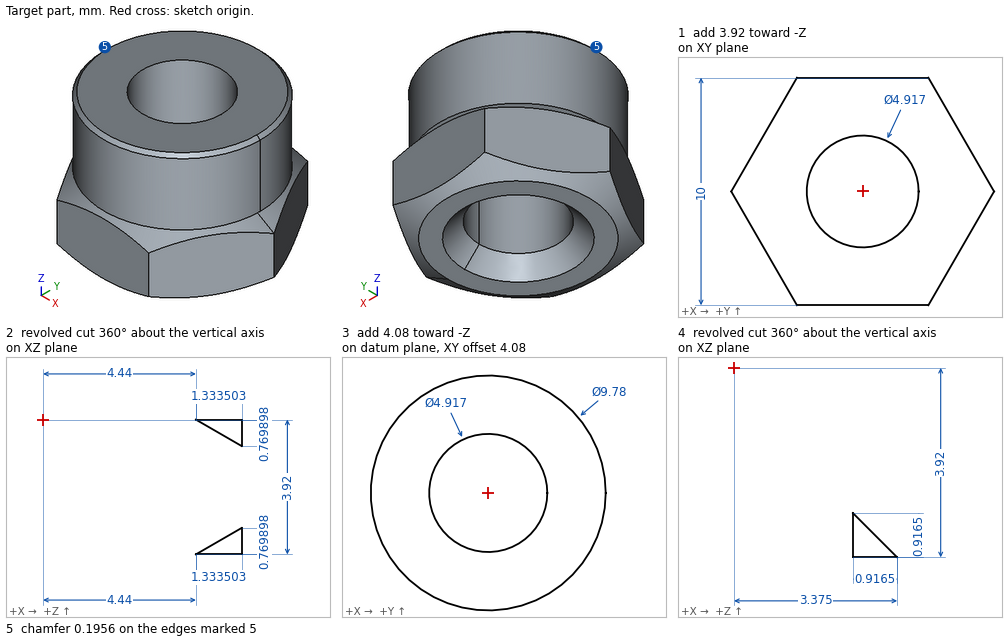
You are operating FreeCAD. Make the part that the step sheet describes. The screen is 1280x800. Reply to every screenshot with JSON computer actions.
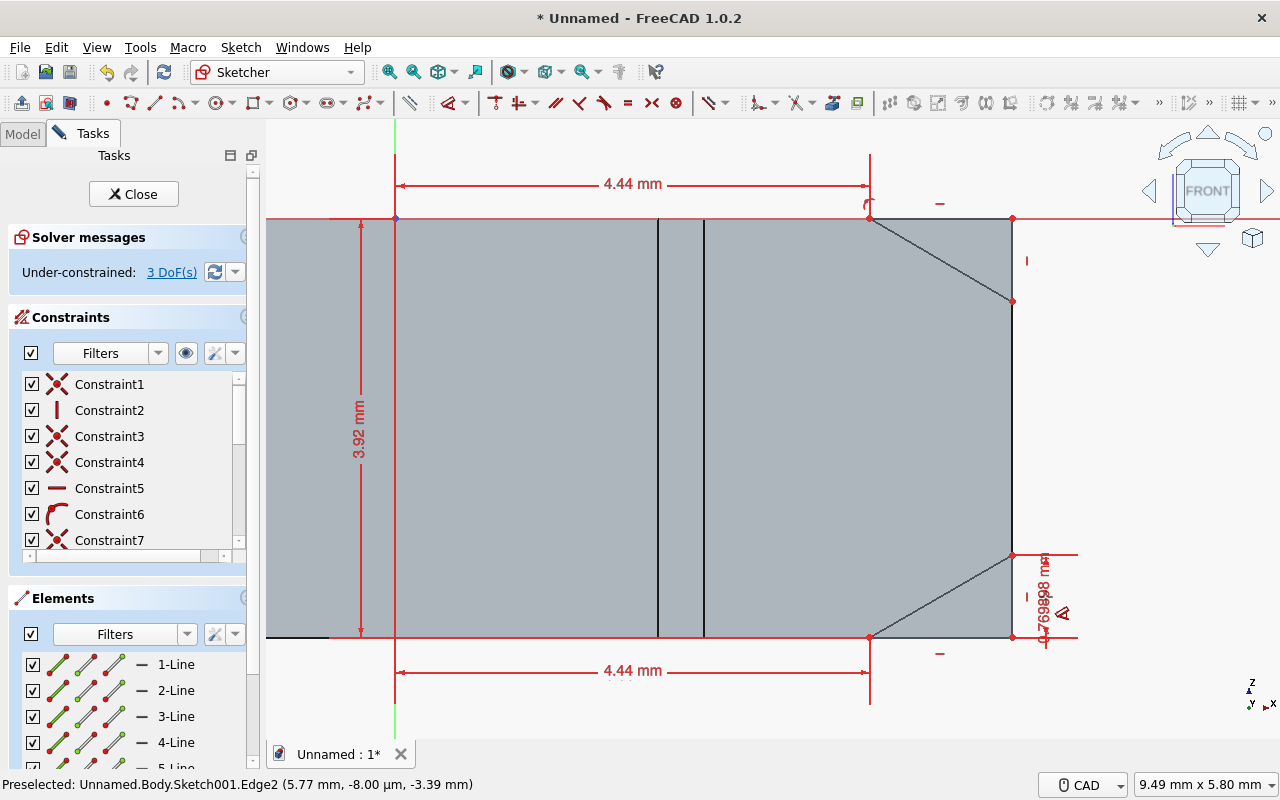
{"action": "left_click", "coordinate": [969, 638]}
{"action": "left_click", "coordinate": [941, 672]}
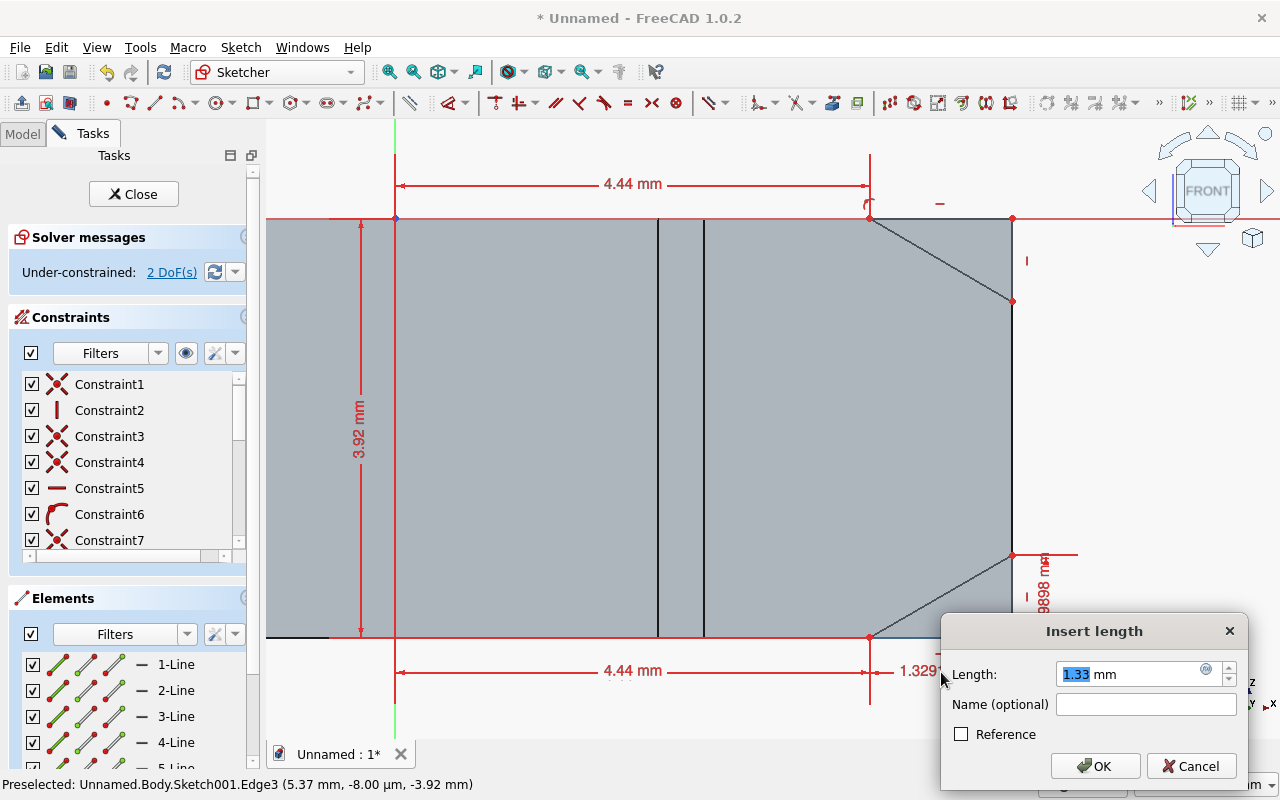
{"action": "type", "text": "1.333503"}
{"action": "key", "text": "Return"}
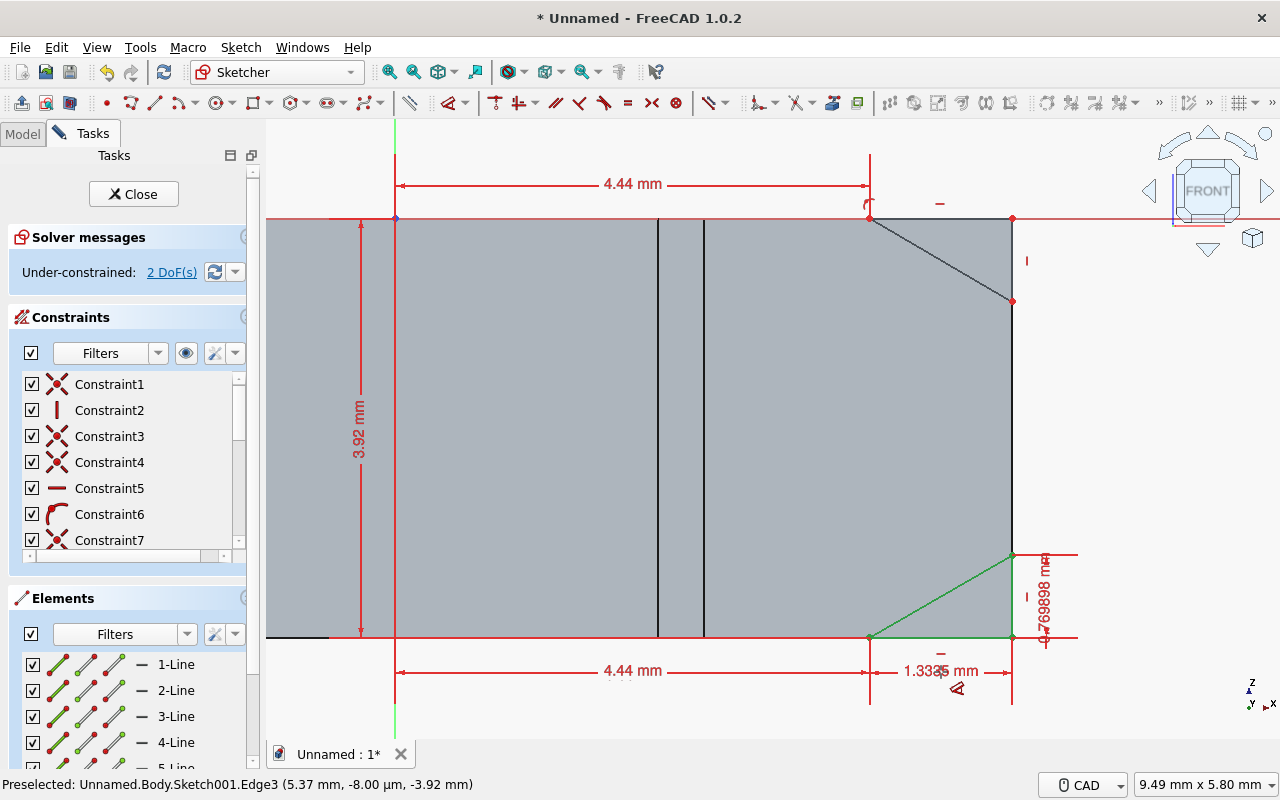
{"action": "left_click", "coordinate": [913, 219]}
{"action": "left_click", "coordinate": [941, 185]}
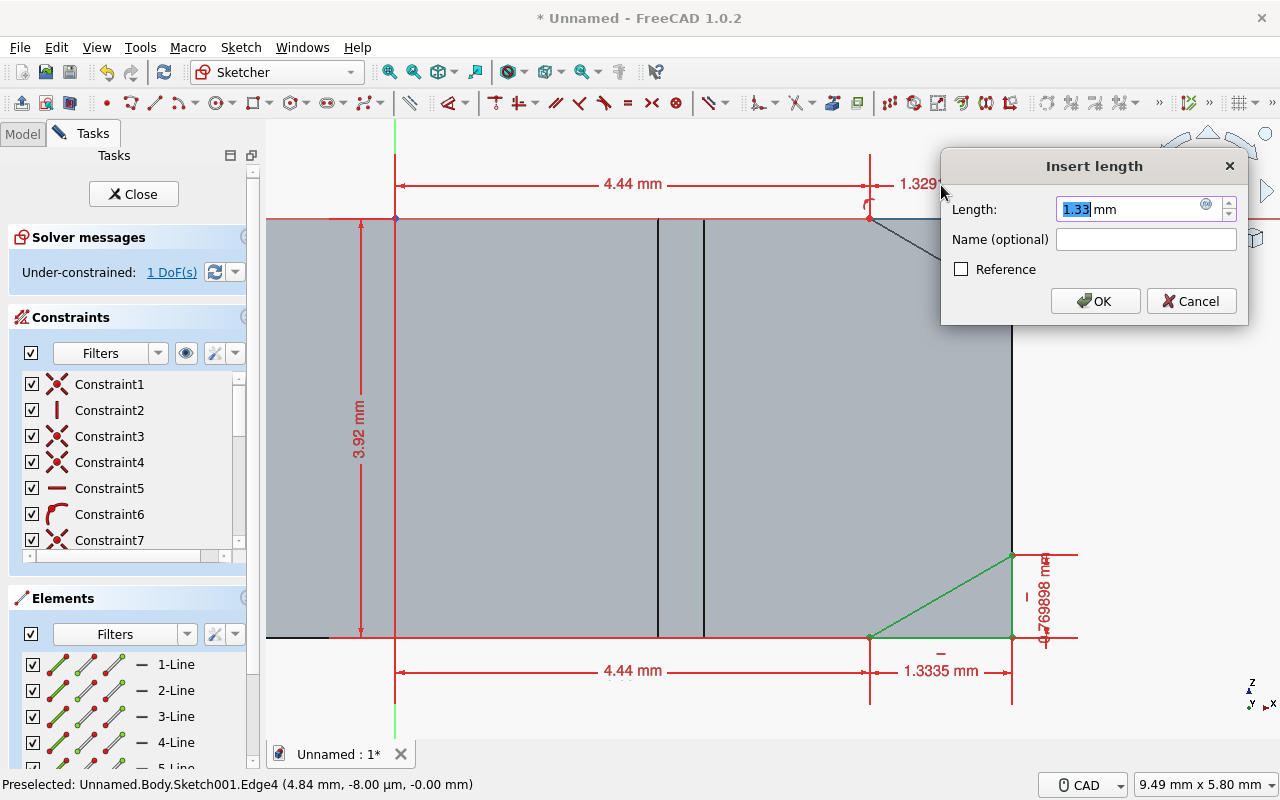
{"action": "type", "text": "1.333503"}
{"action": "key", "text": "Return"}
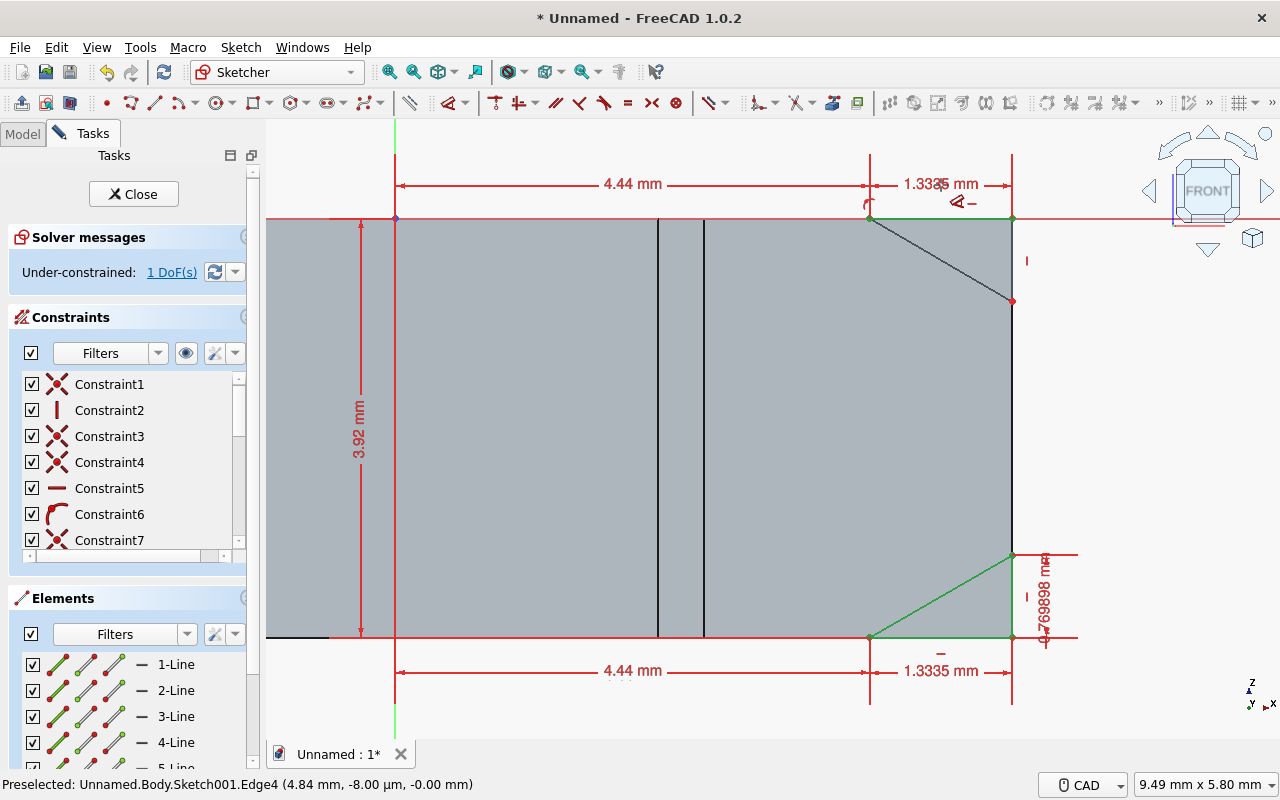
{"action": "left_click", "coordinate": [1012, 244]}
{"action": "left_click", "coordinate": [1046, 260]}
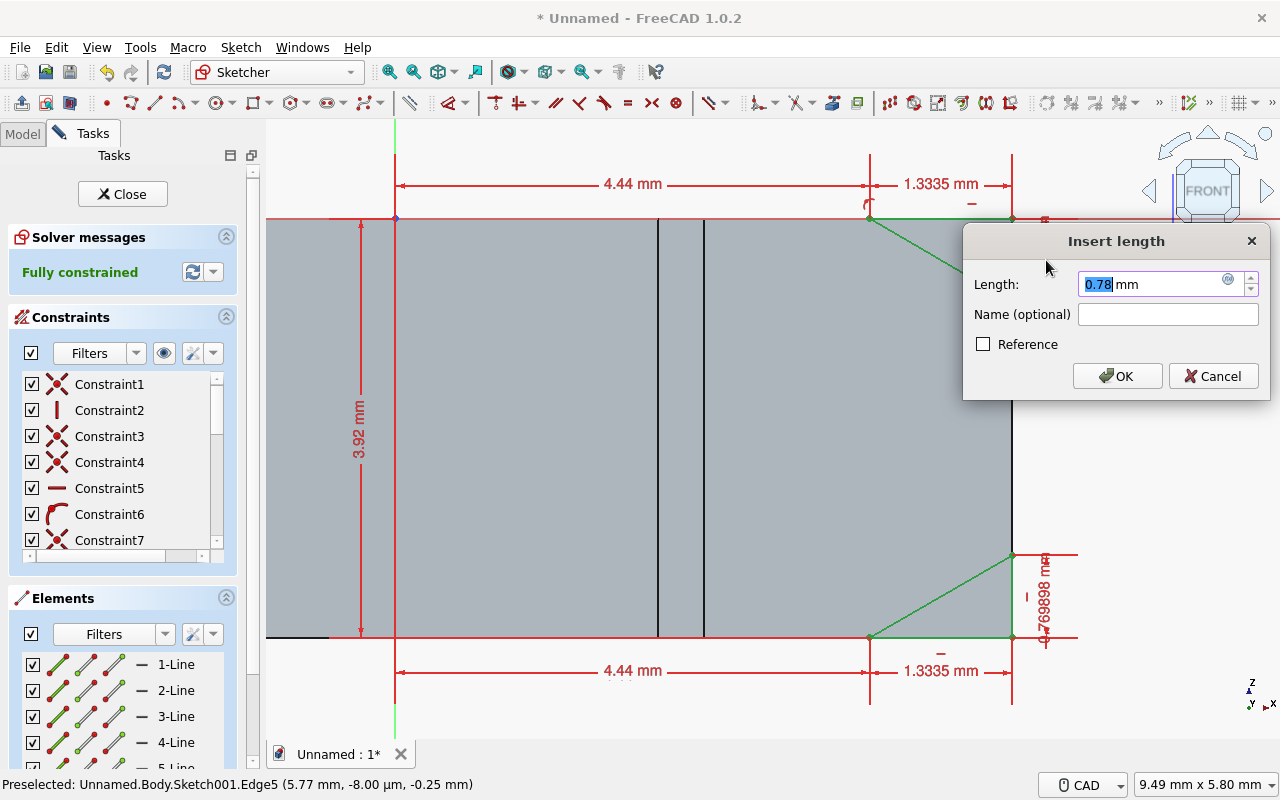
{"action": "type", "text": "0.769898"}
{"action": "key", "text": "Return"}
{"action": "key", "text": "Escape"}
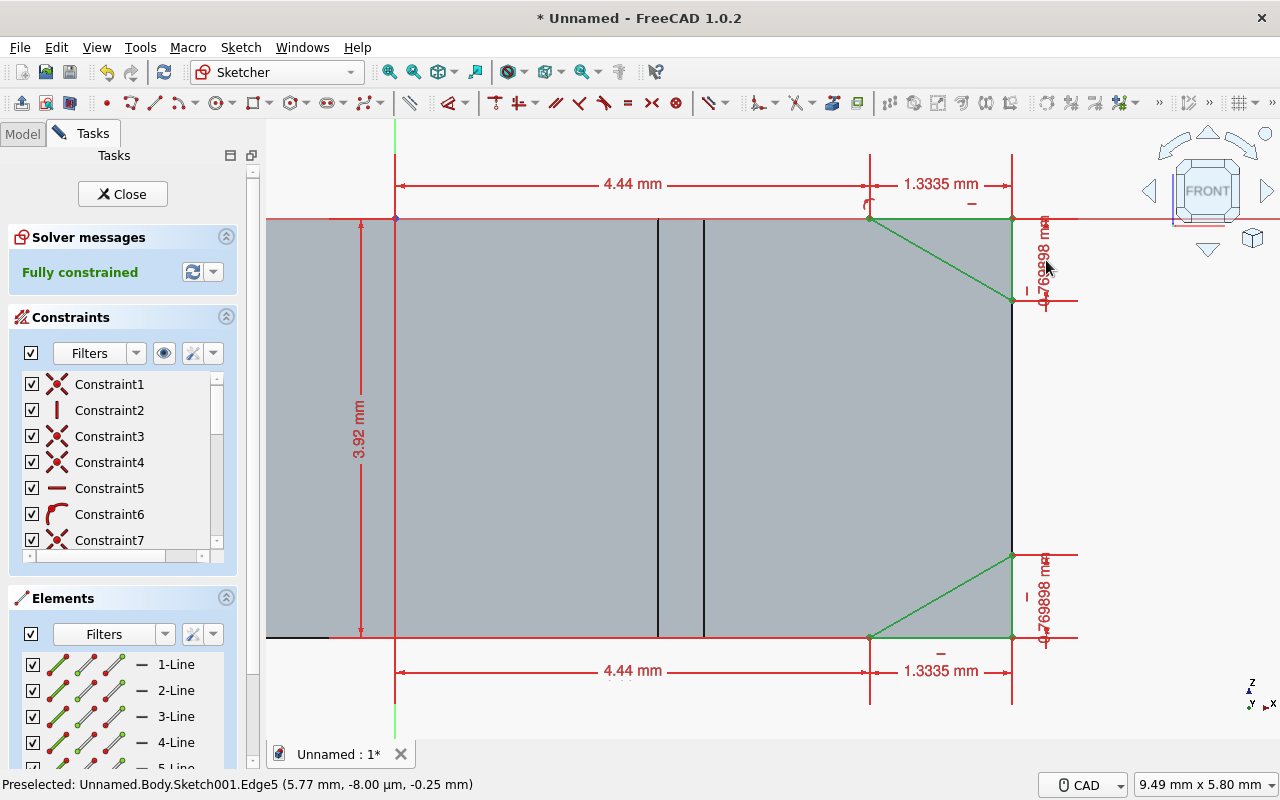
{"action": "left_click", "coordinate": [123, 194]}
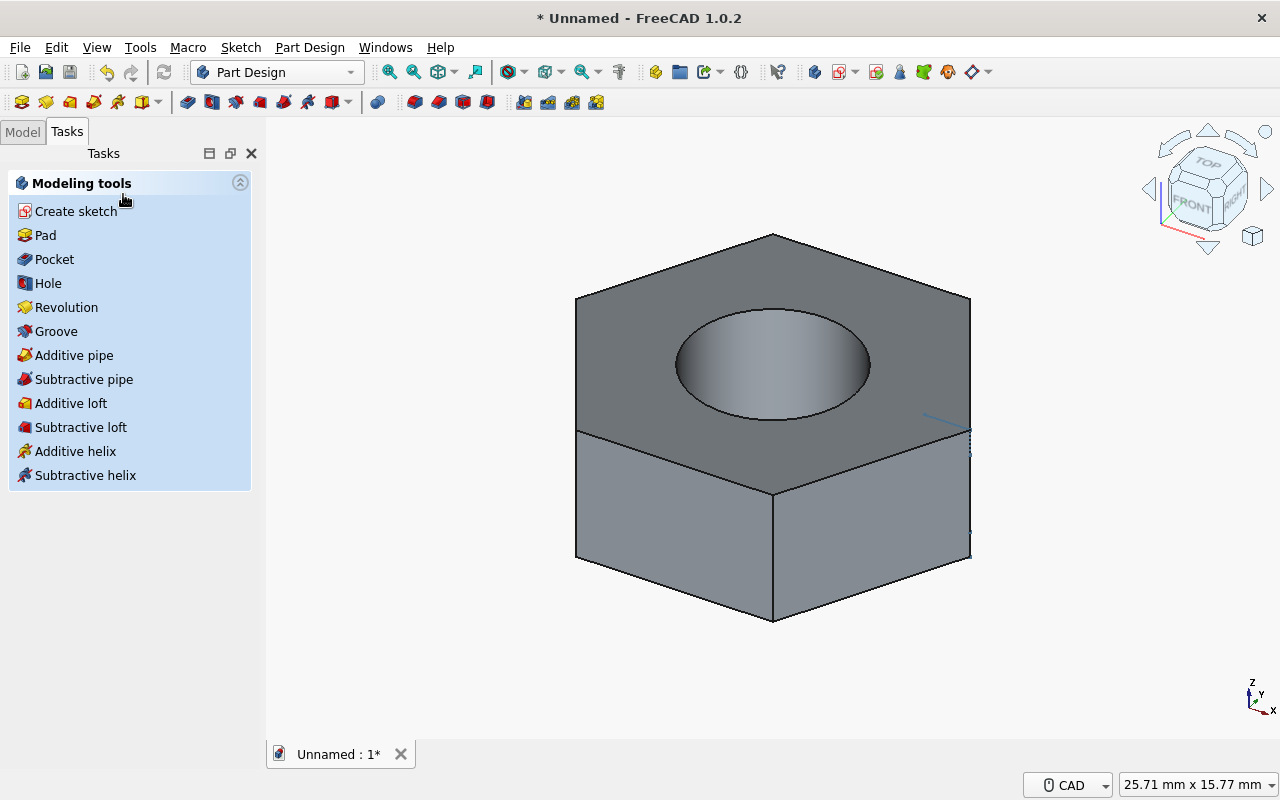
{"action": "left_click", "coordinate": [236, 102]}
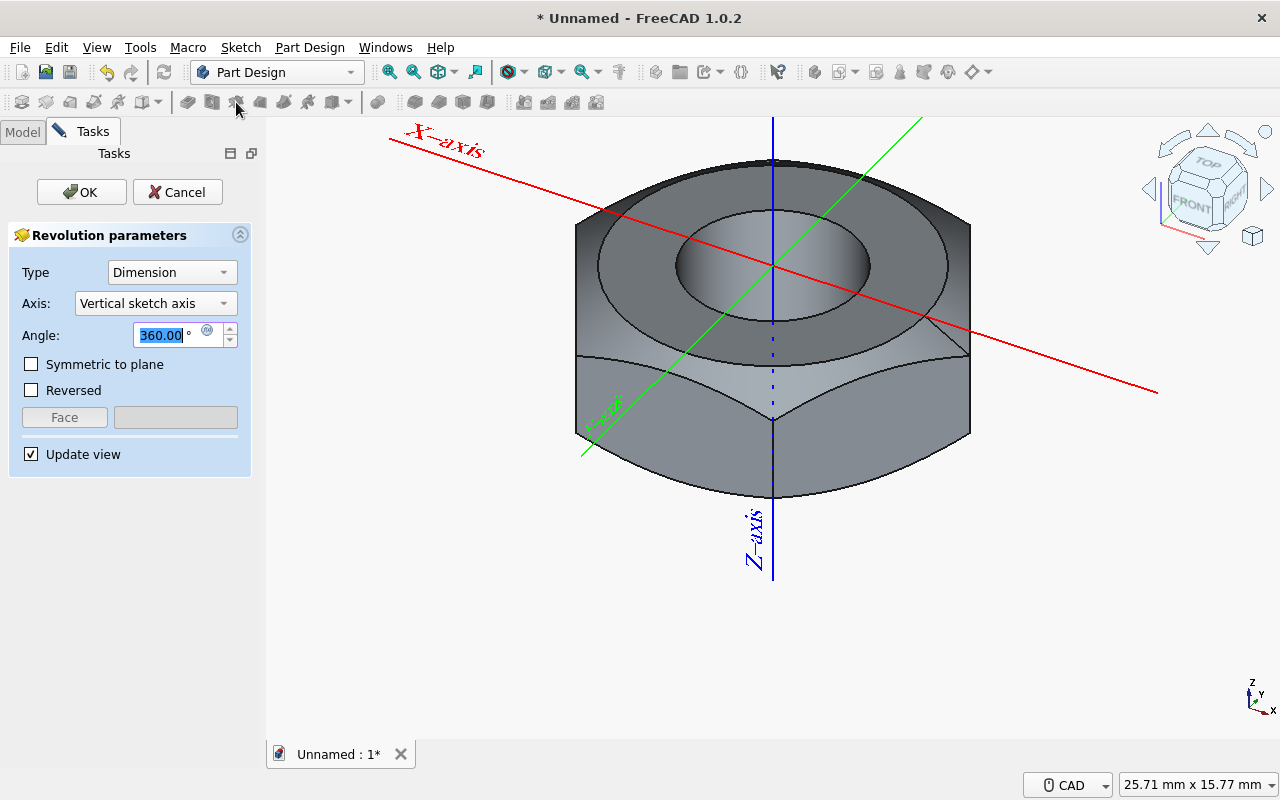
{"action": "left_click", "coordinate": [82, 192]}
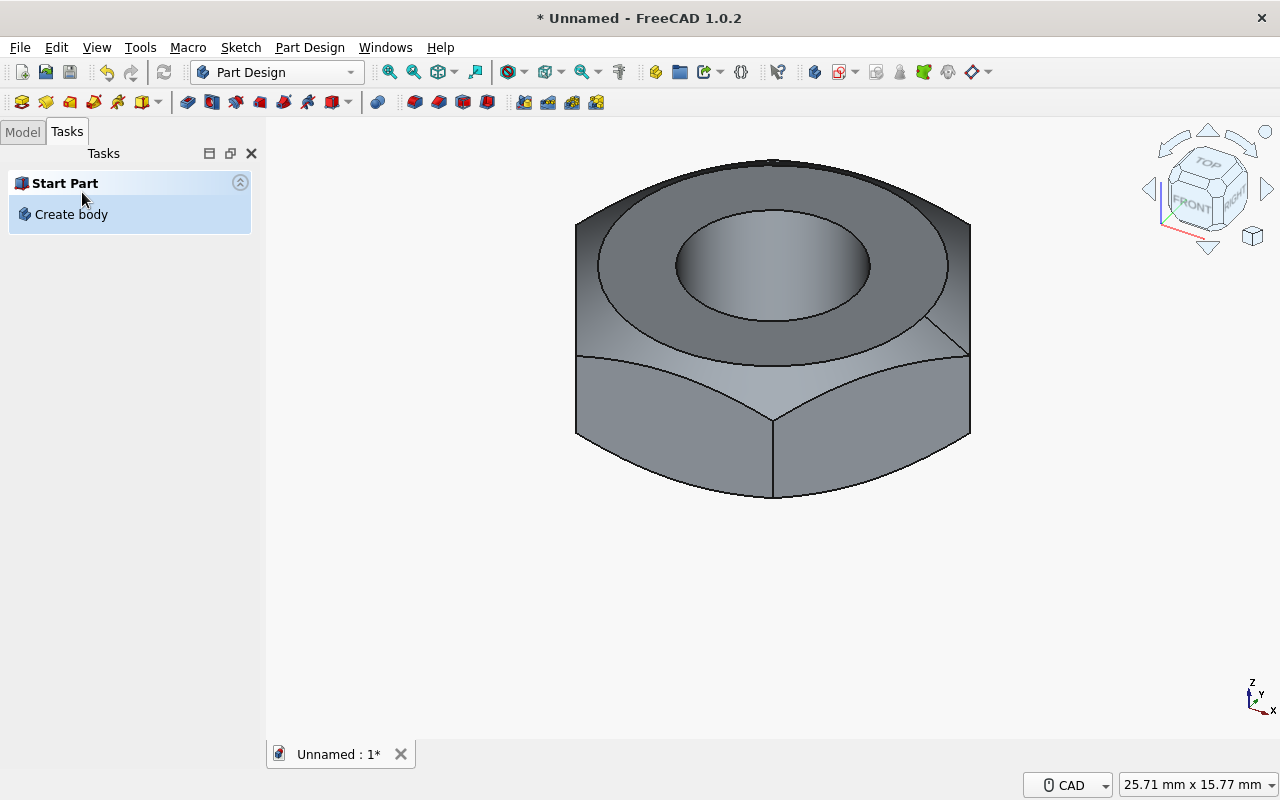
{"action": "key", "text": "v f"}